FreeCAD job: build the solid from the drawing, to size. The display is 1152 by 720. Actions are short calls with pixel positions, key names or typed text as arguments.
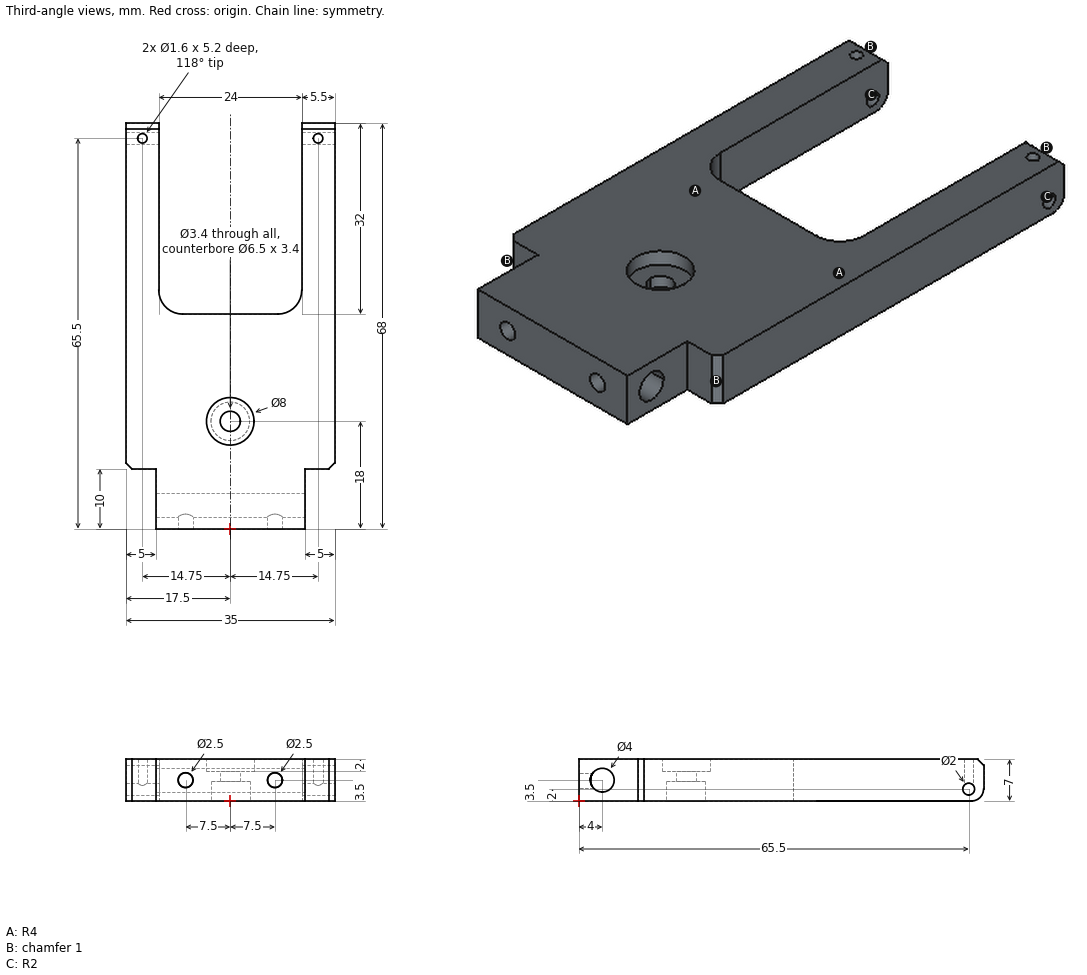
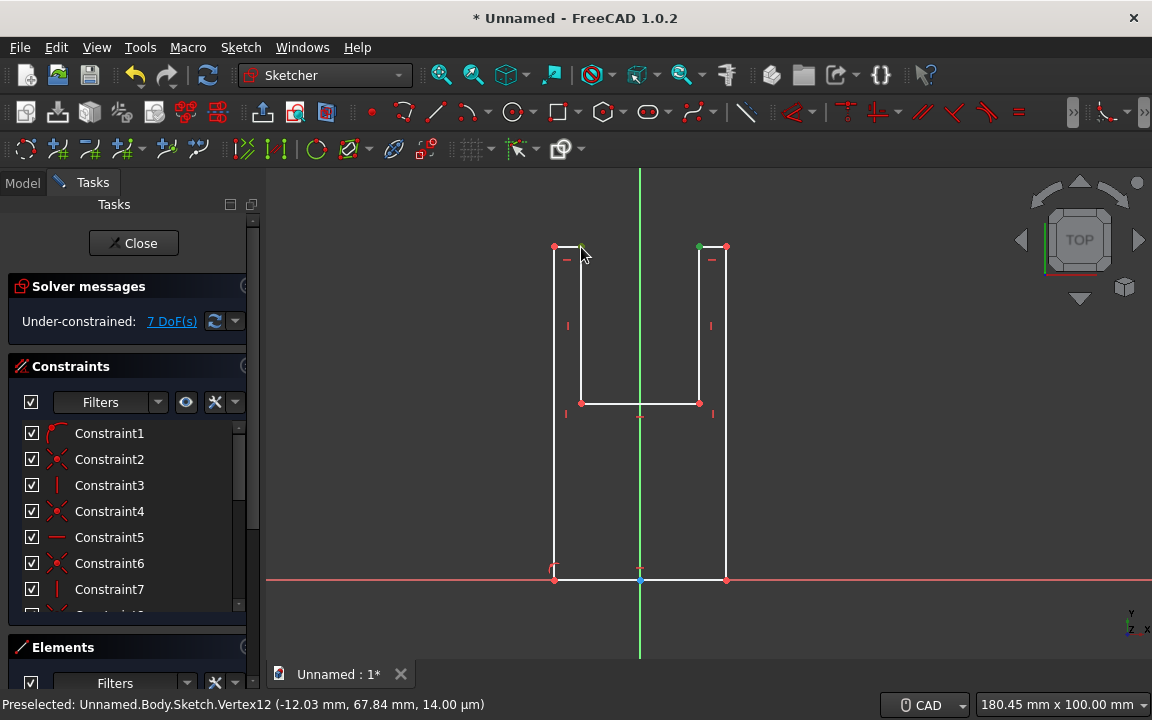
click(640, 538)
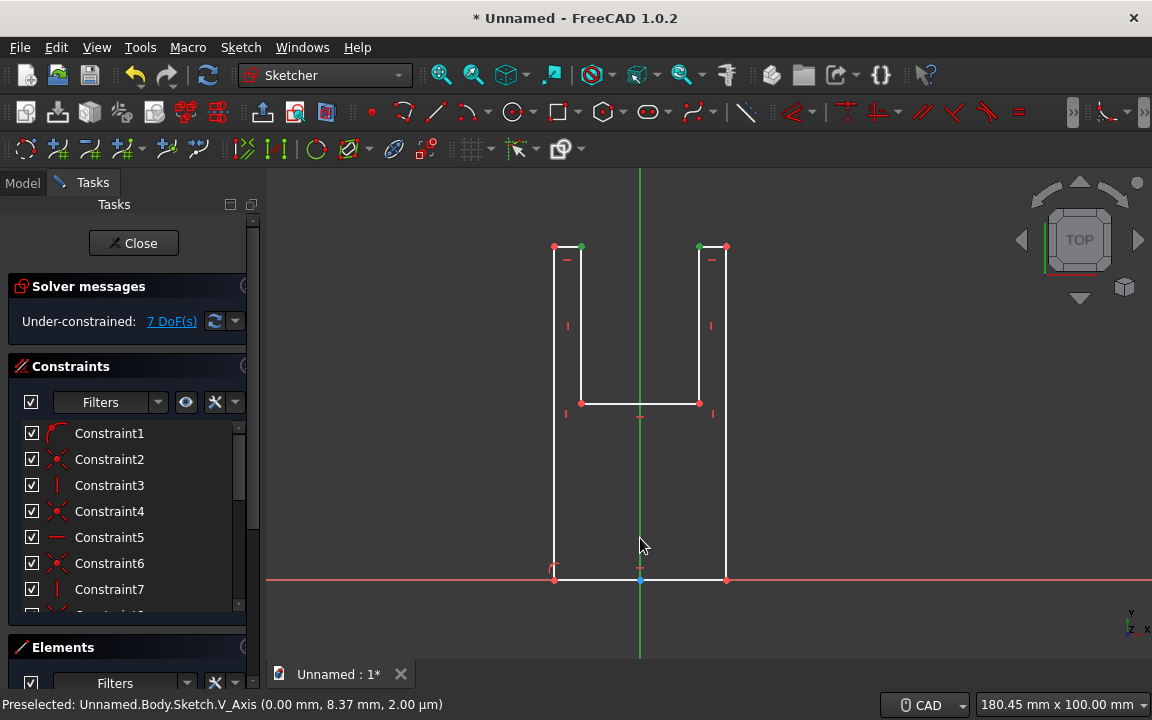
key(s)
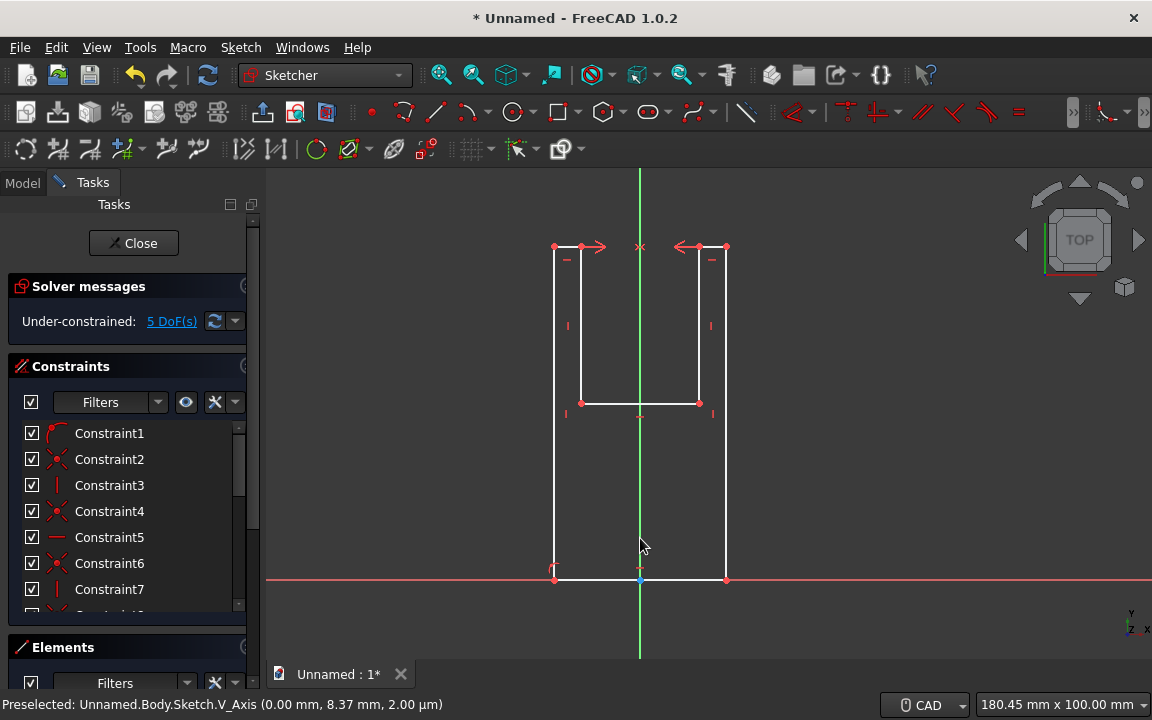
click(792, 112)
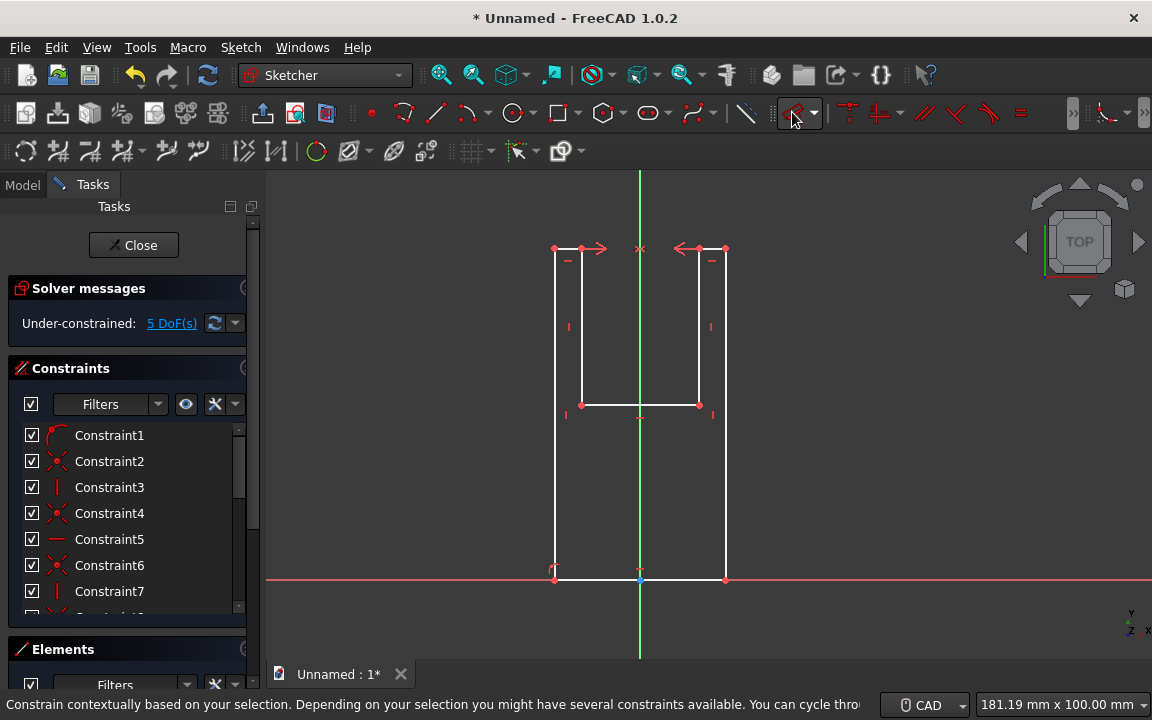
click(606, 580)
click(601, 614)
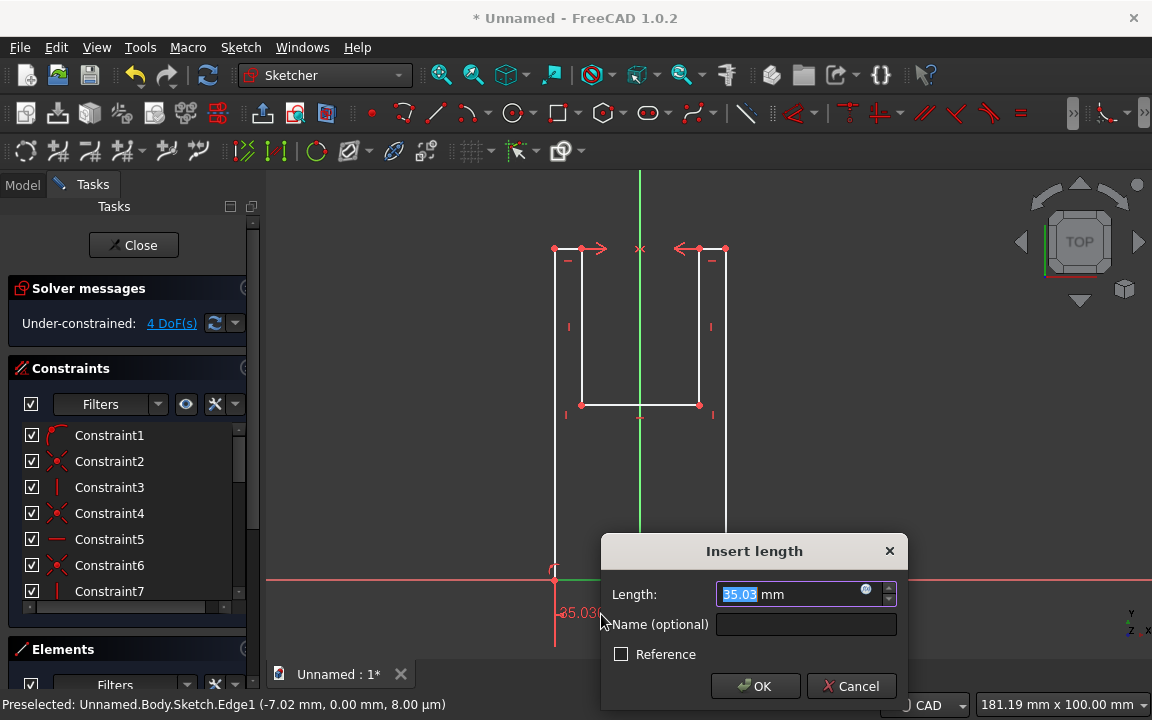
text(35)
key(Return)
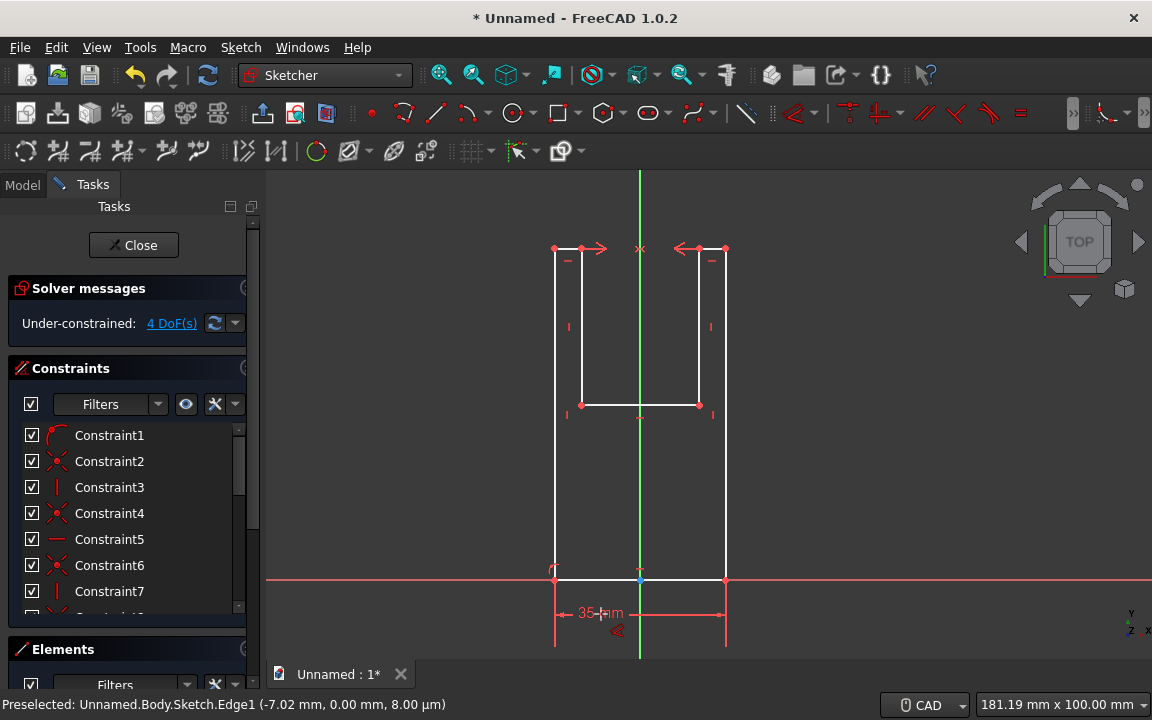
click(726, 481)
click(760, 415)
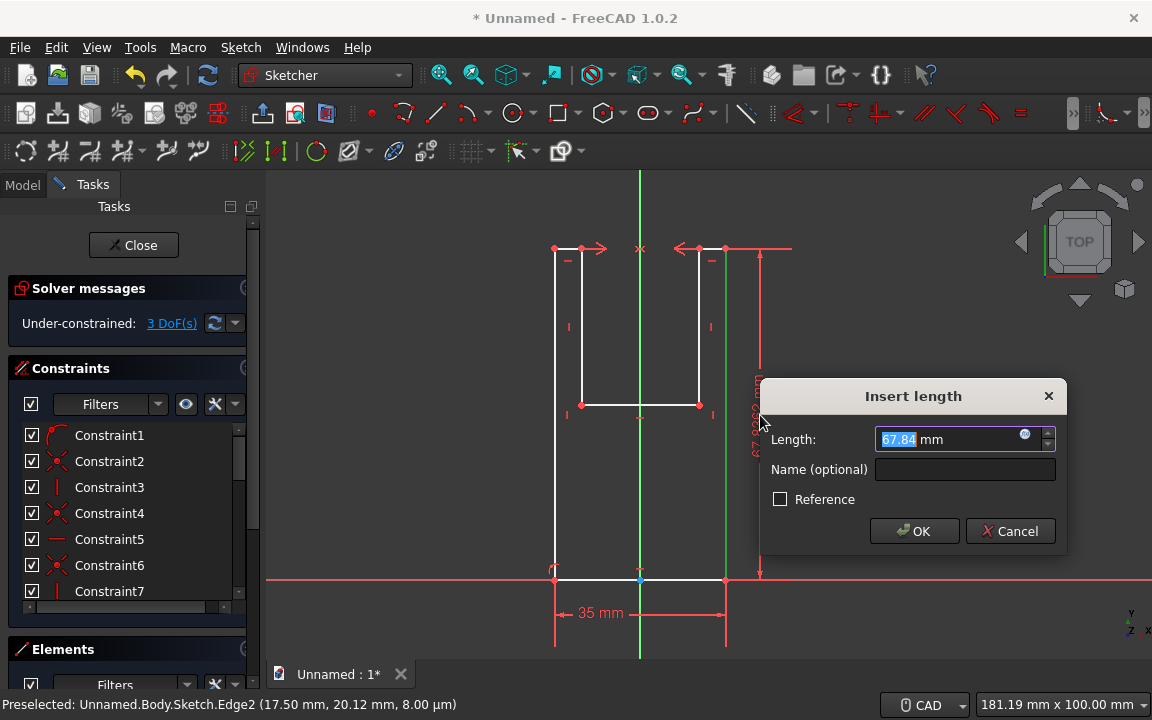
text(68)
key(Return)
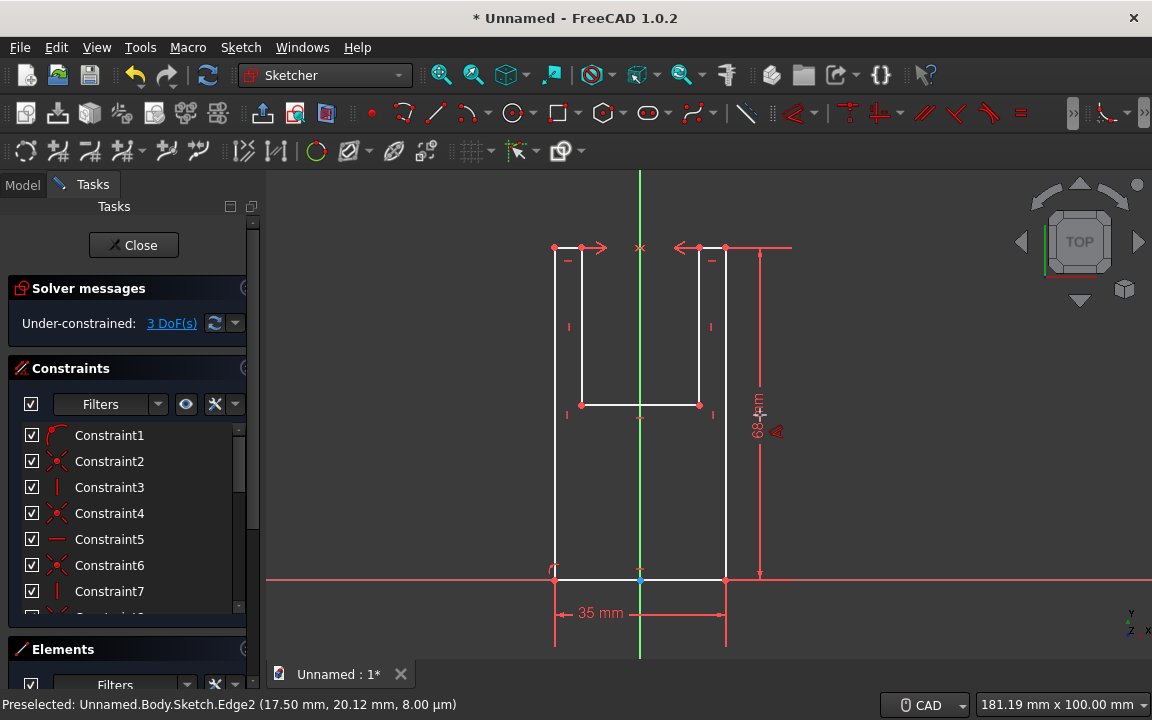
click(699, 295)
click(665, 326)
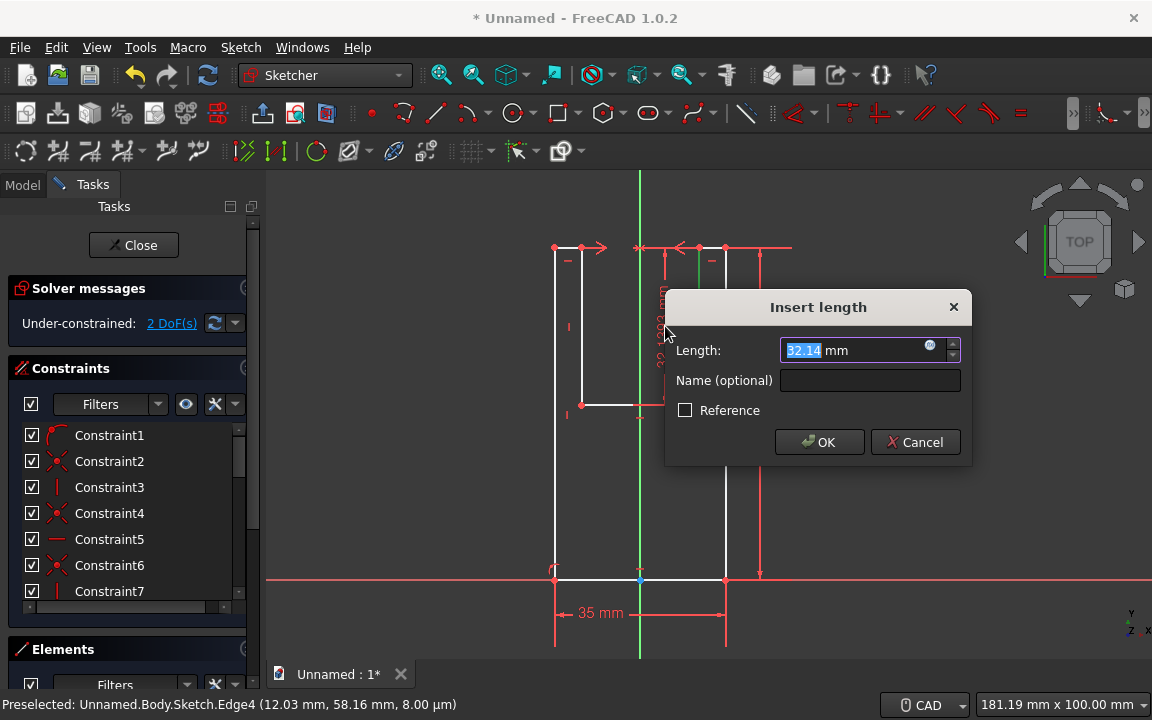
text(32)
key(Return)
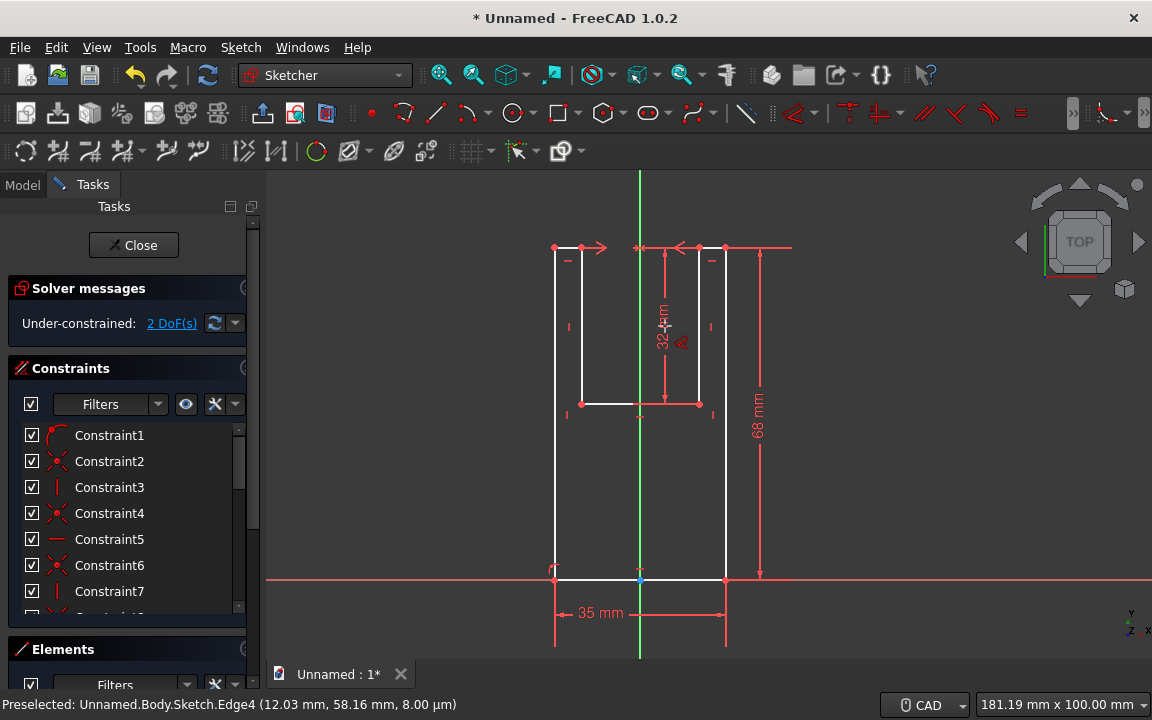
click(664, 404)
click(613, 370)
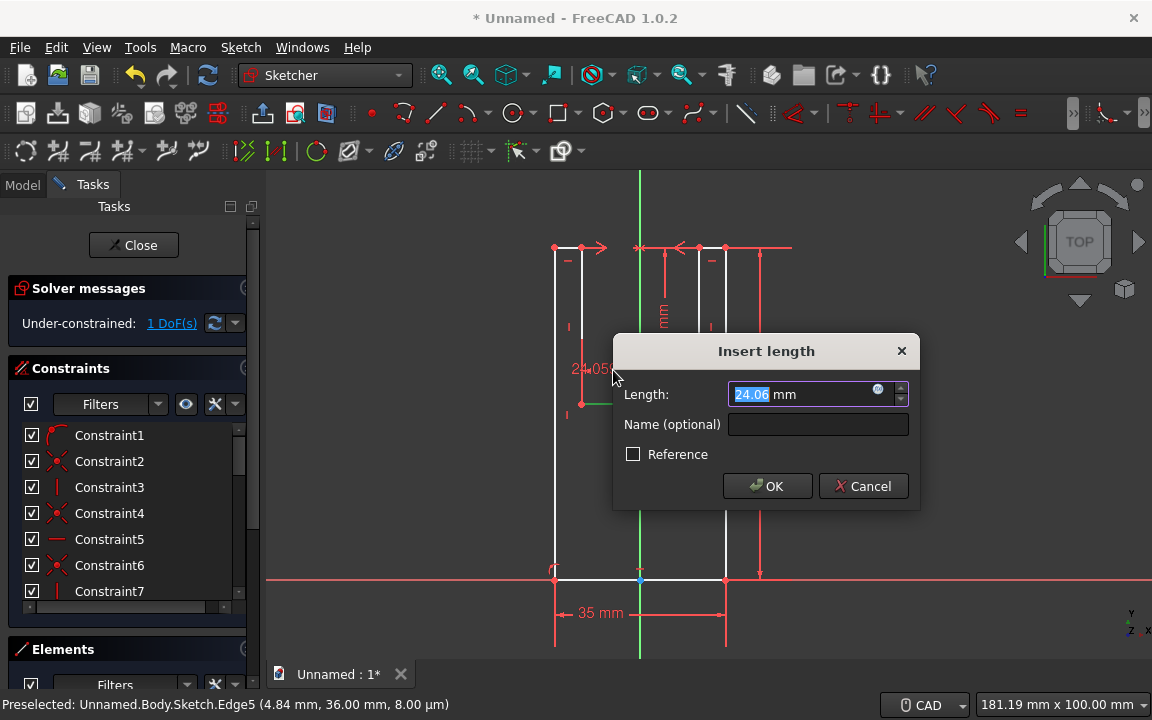
text(24)
key(Return)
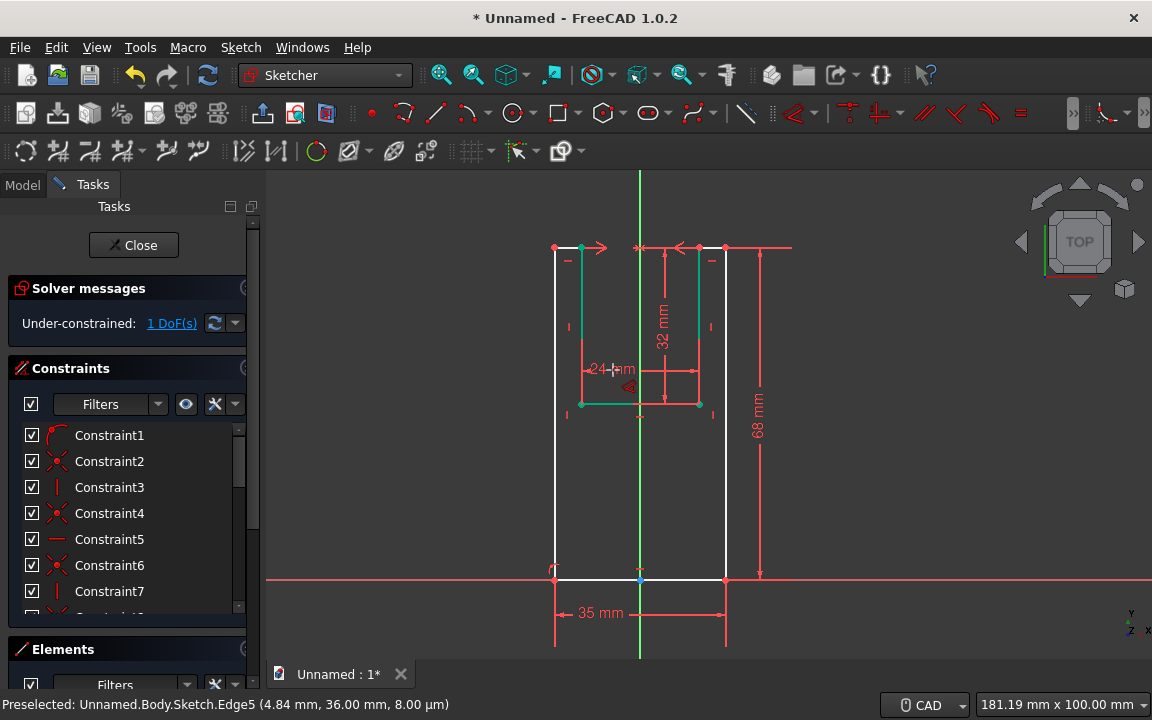
scroll(715, 248, up, 2)